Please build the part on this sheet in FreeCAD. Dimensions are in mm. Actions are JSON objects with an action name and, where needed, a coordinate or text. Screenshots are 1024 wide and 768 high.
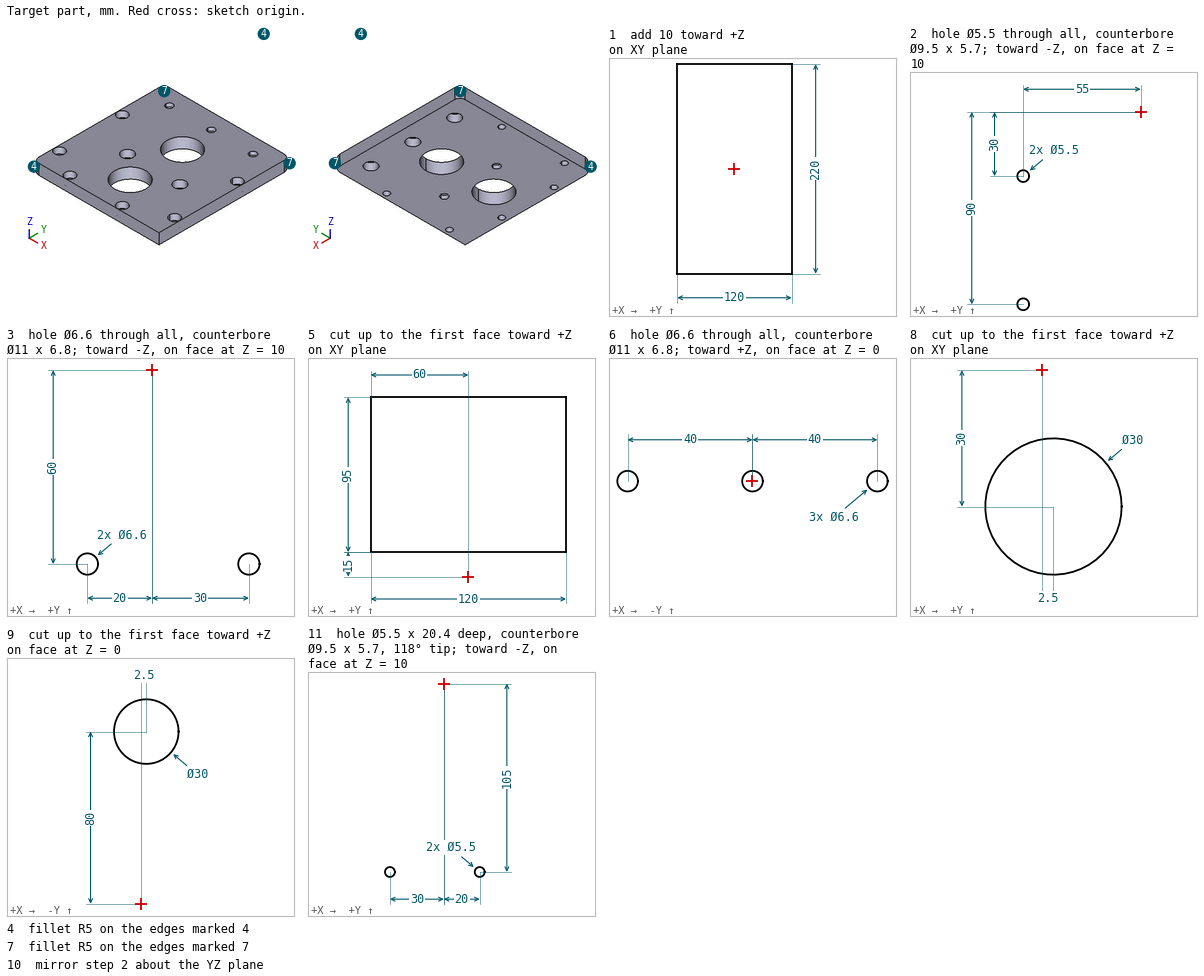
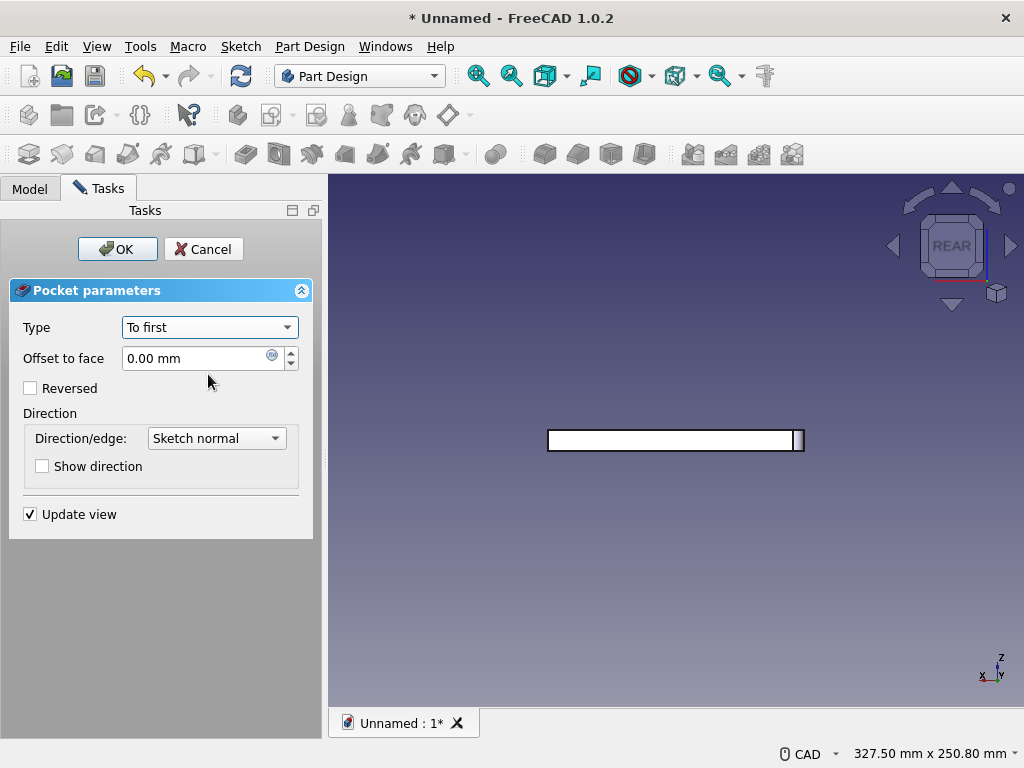
{"action": "left_click", "coordinate": [31, 388]}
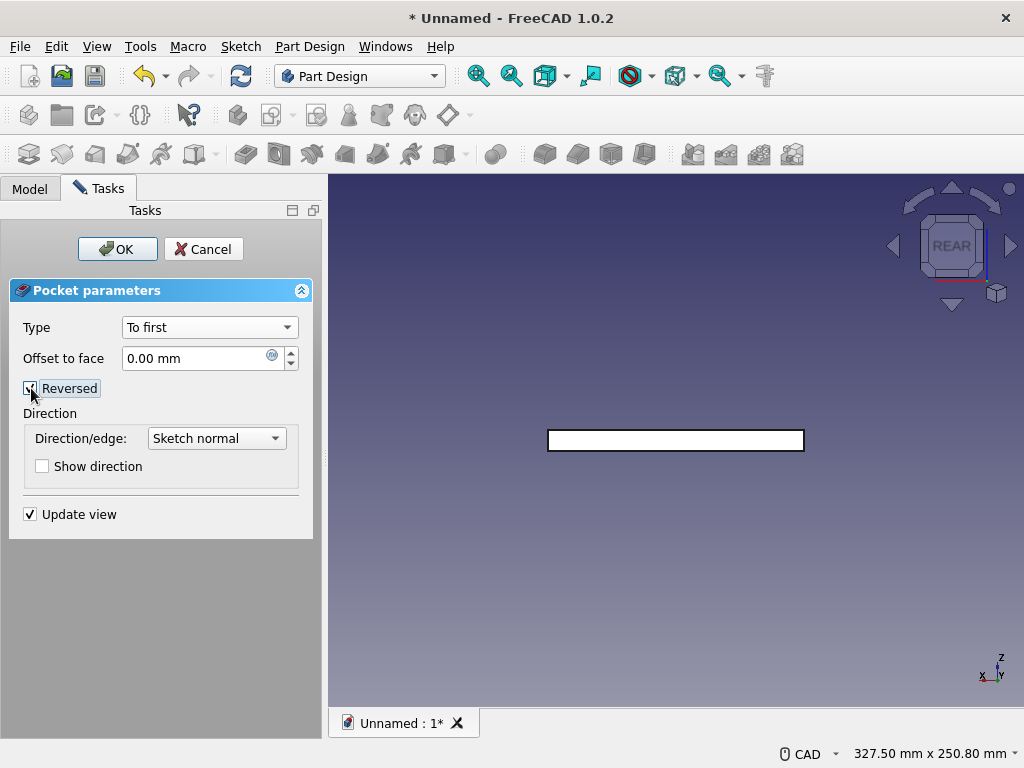
{"action": "left_click", "coordinate": [118, 249]}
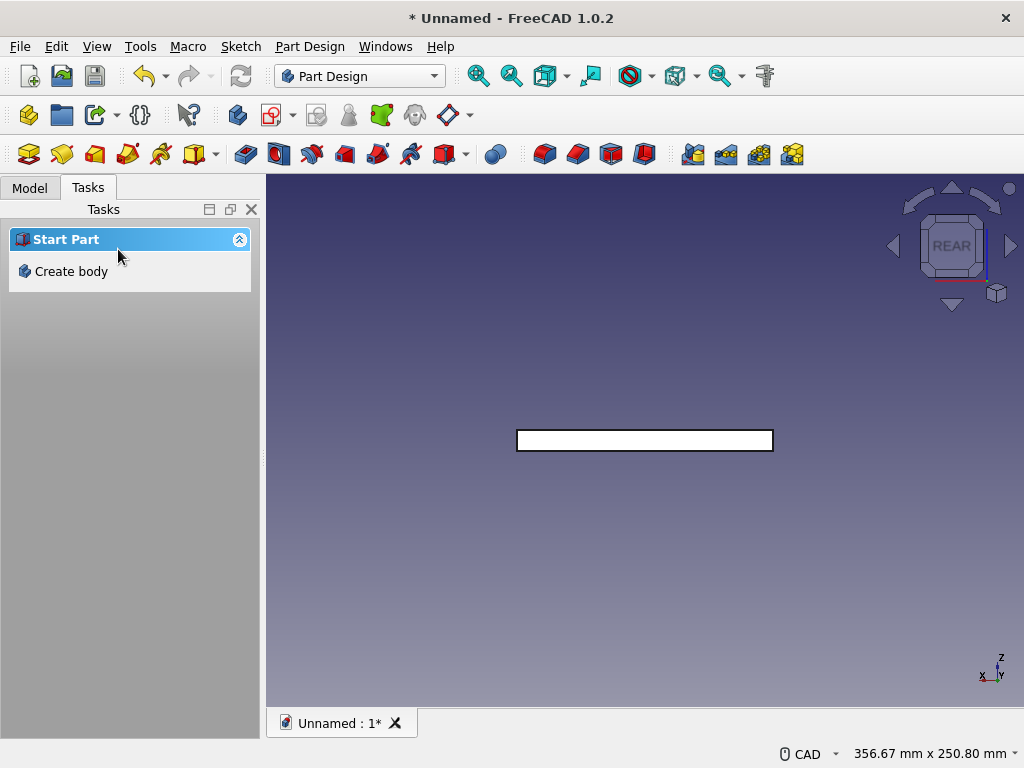
{"action": "left_click", "coordinate": [479, 76]}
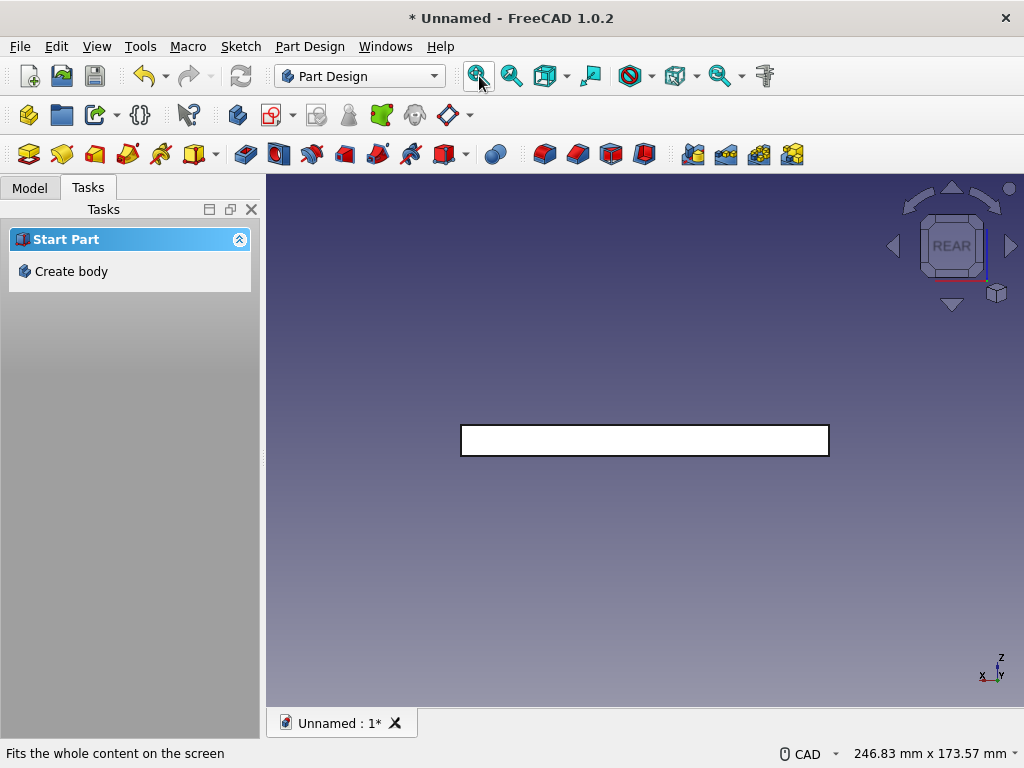
{"action": "key", "text": "5"}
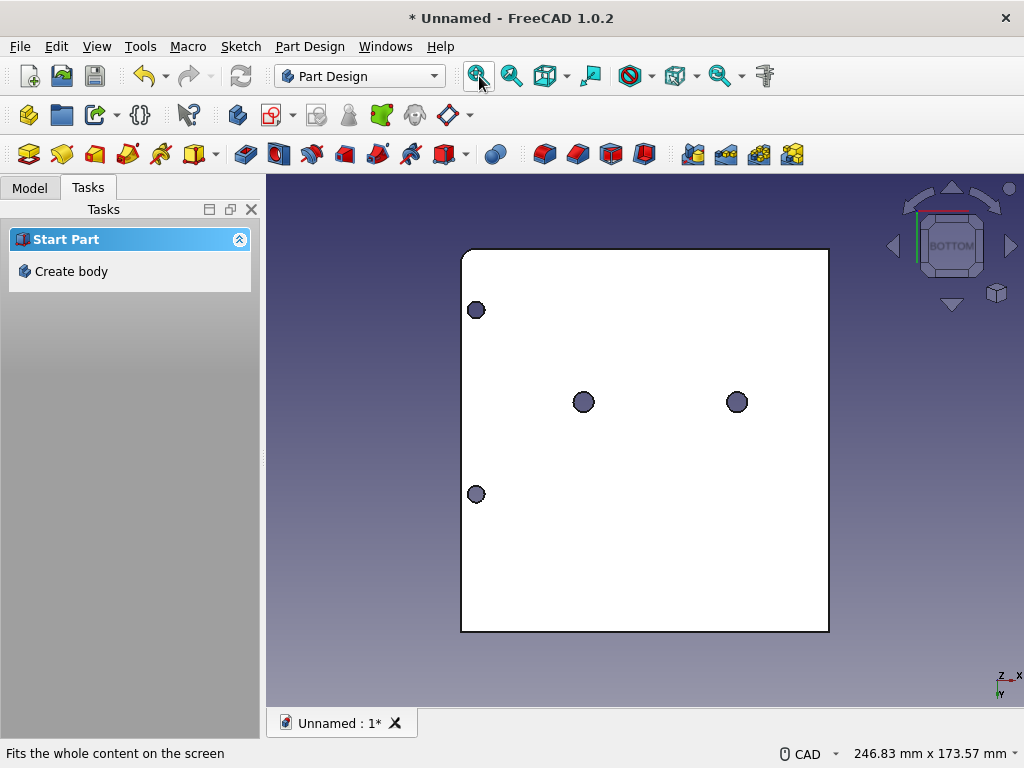
{"action": "left_click", "coordinate": [645, 494]}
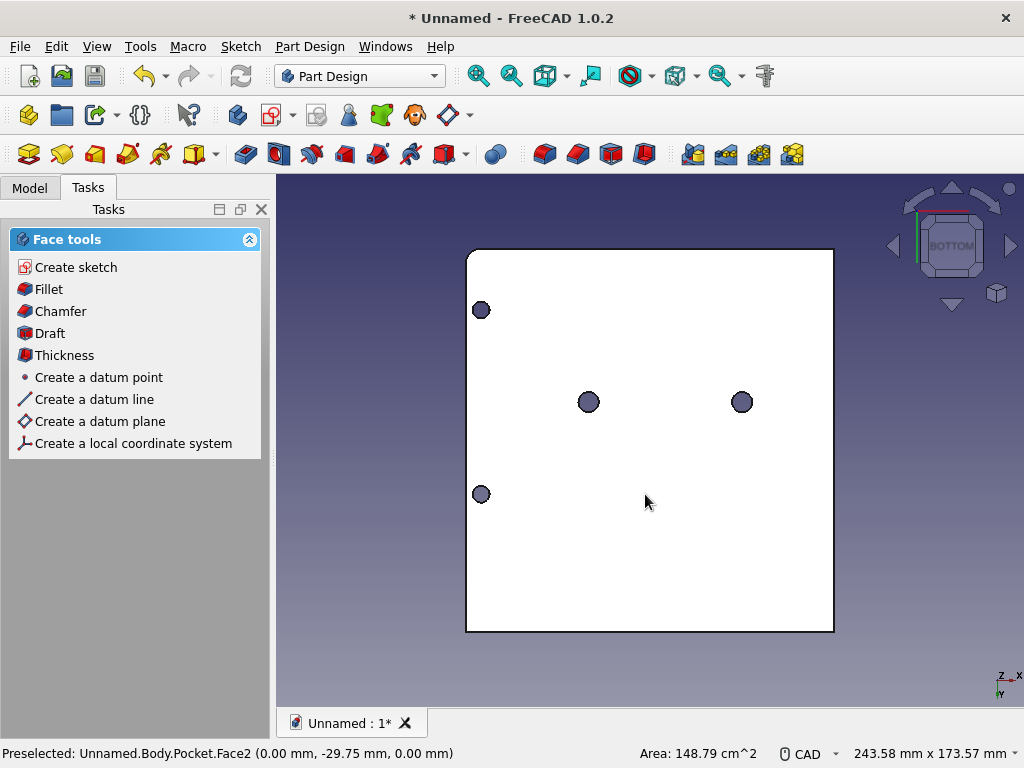
{"action": "left_click", "coordinate": [270, 116]}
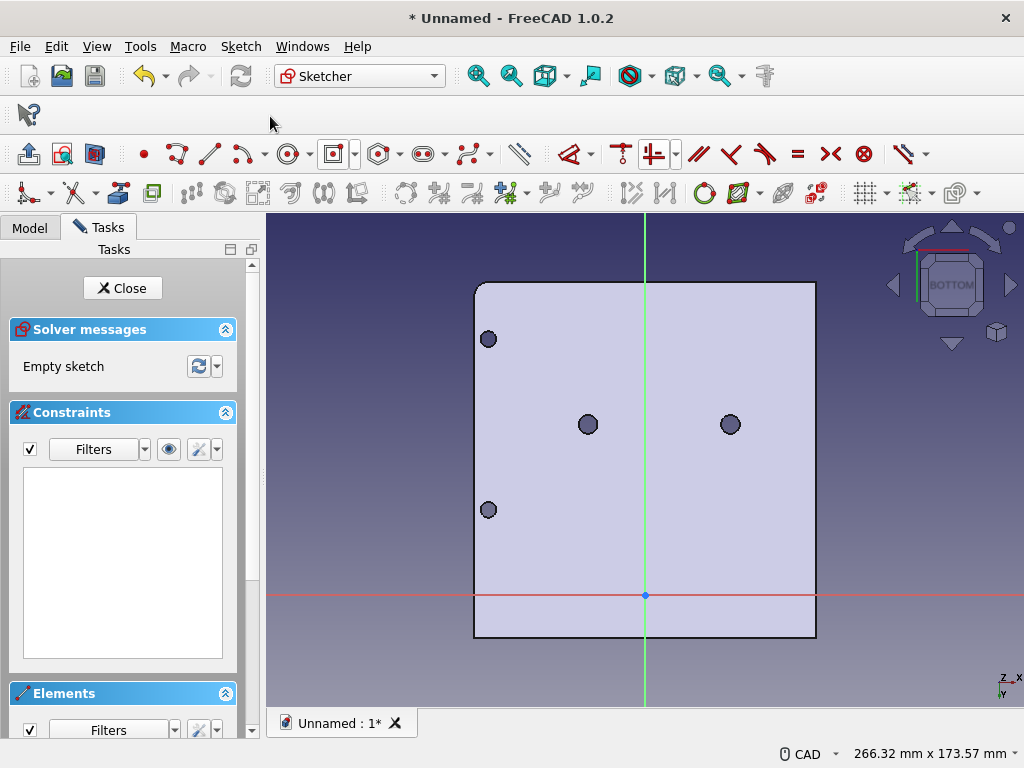
{"action": "scroll", "coordinate": [784, 679], "scroll_direction": "up", "scroll_amount": 2}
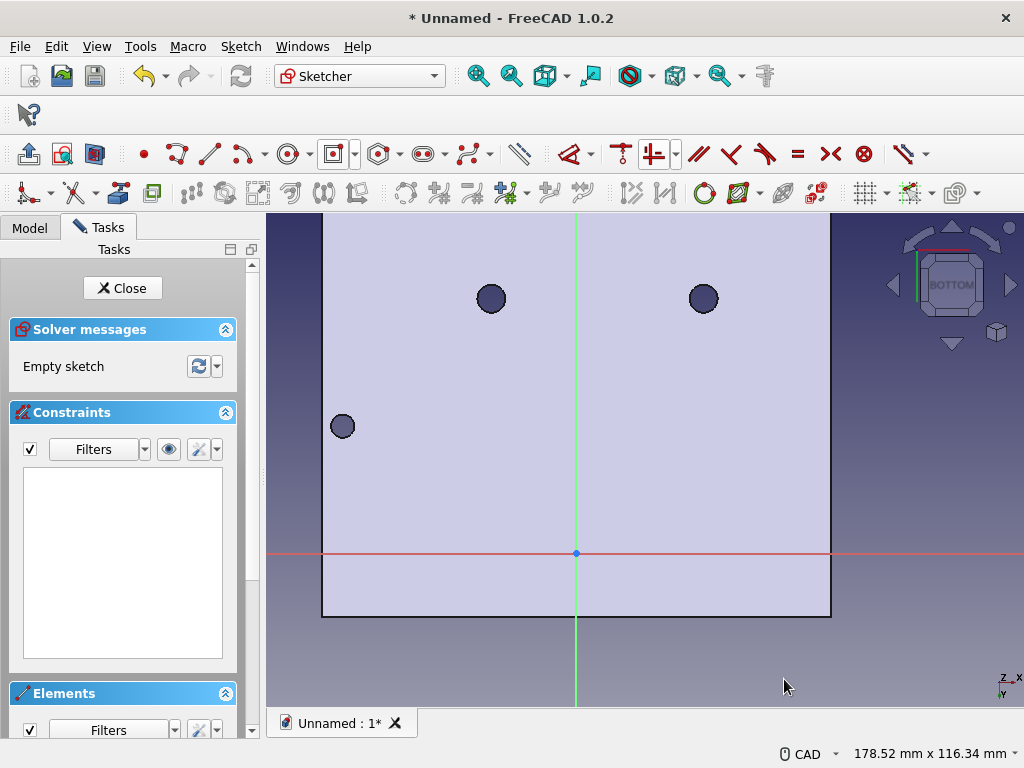
{"action": "left_click", "coordinate": [288, 154]}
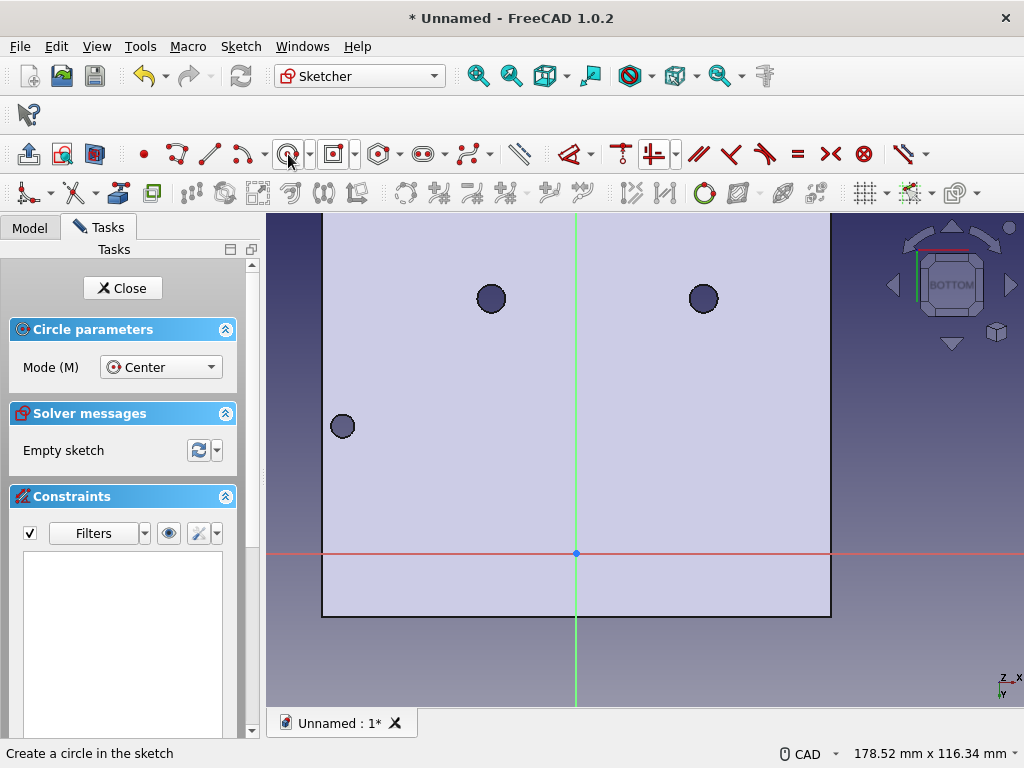
{"action": "scroll", "coordinate": [746, 554], "scroll_direction": "up", "scroll_amount": 3}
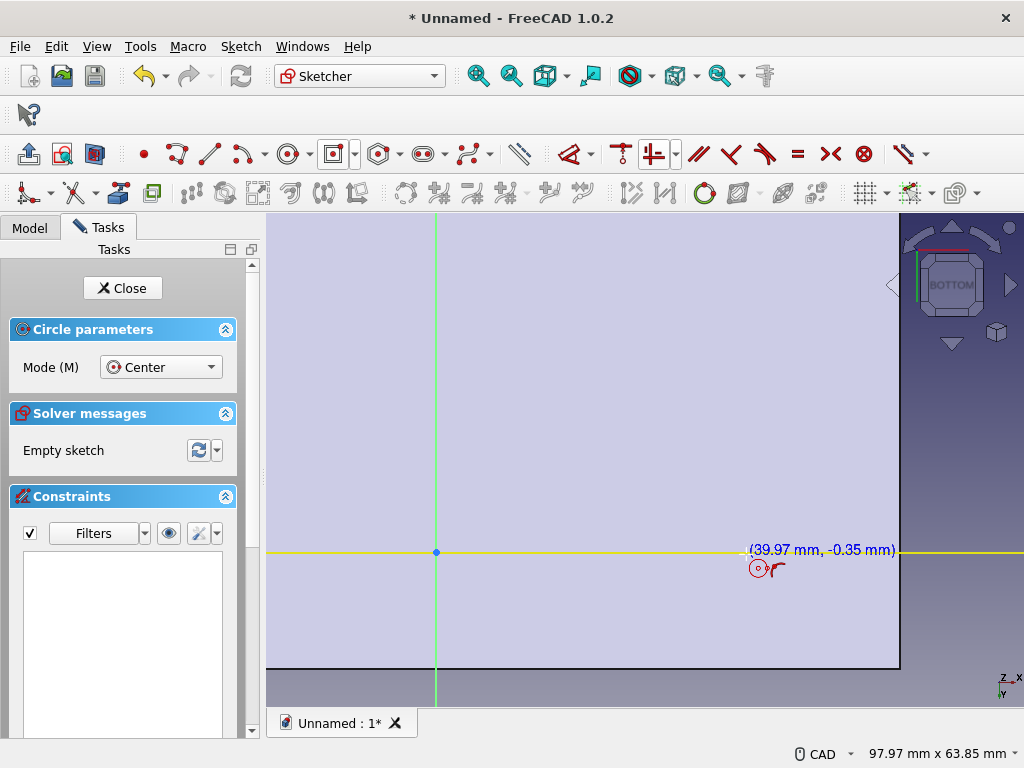
{"action": "left_click", "coordinate": [746, 553]}
{"action": "left_click", "coordinate": [764, 534]}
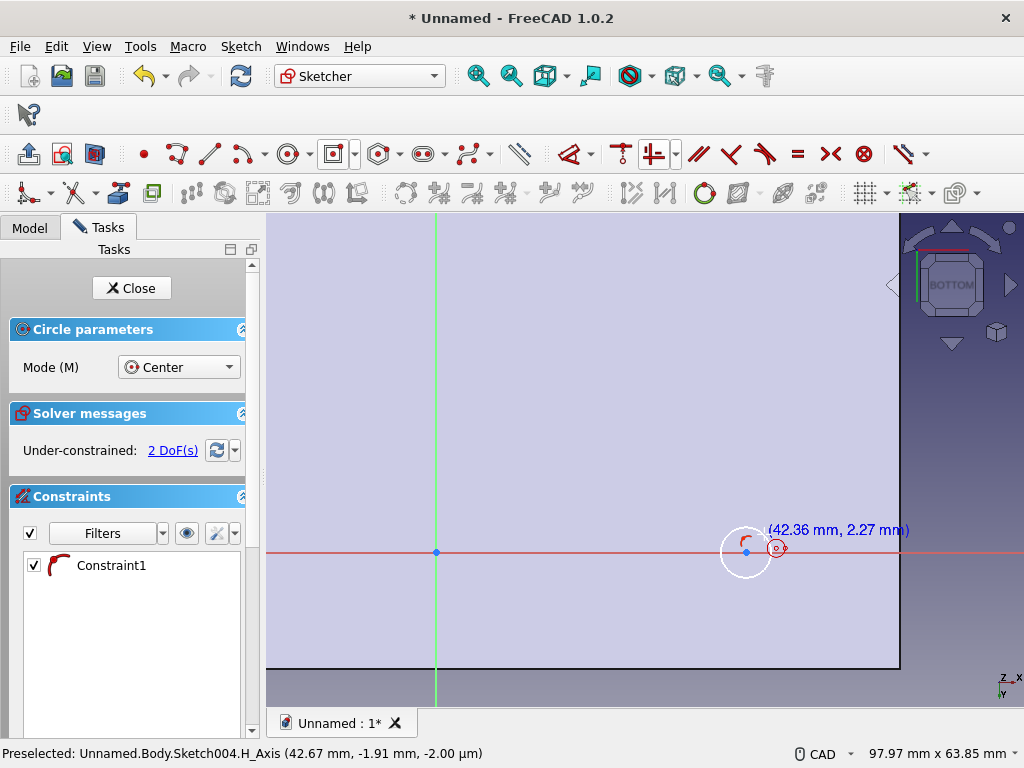
{"action": "left_click", "coordinate": [436, 553]}
{"action": "left_click", "coordinate": [454, 534]}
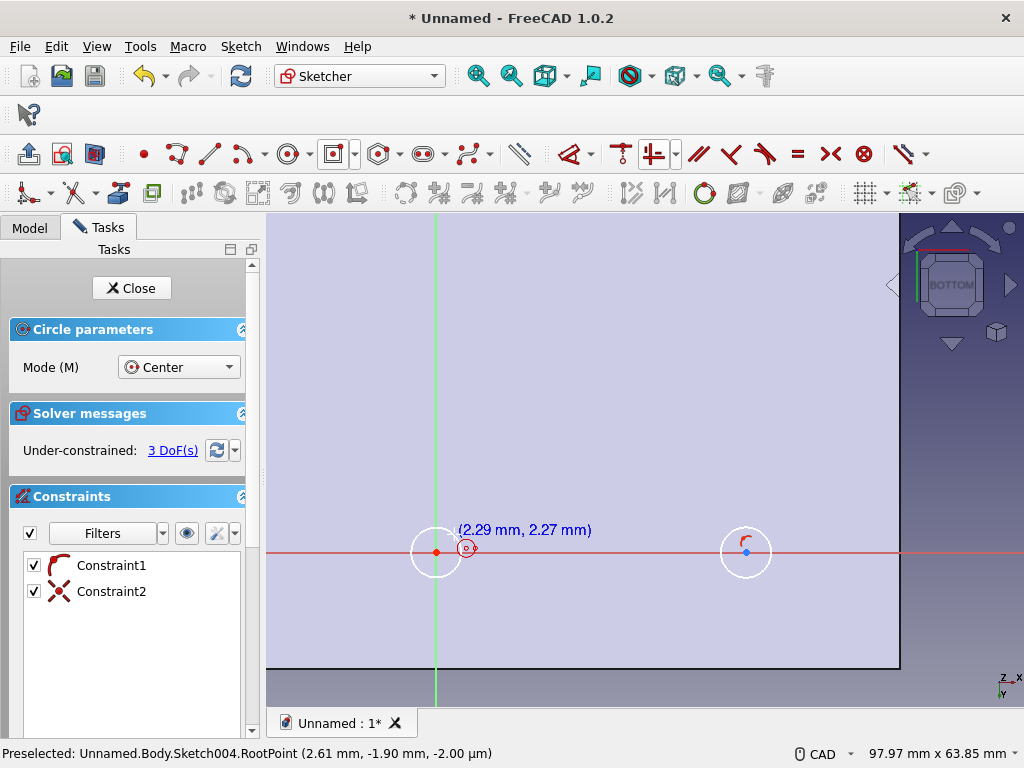
{"action": "scroll", "coordinate": [747, 347], "scroll_direction": "down", "scroll_amount": 3}